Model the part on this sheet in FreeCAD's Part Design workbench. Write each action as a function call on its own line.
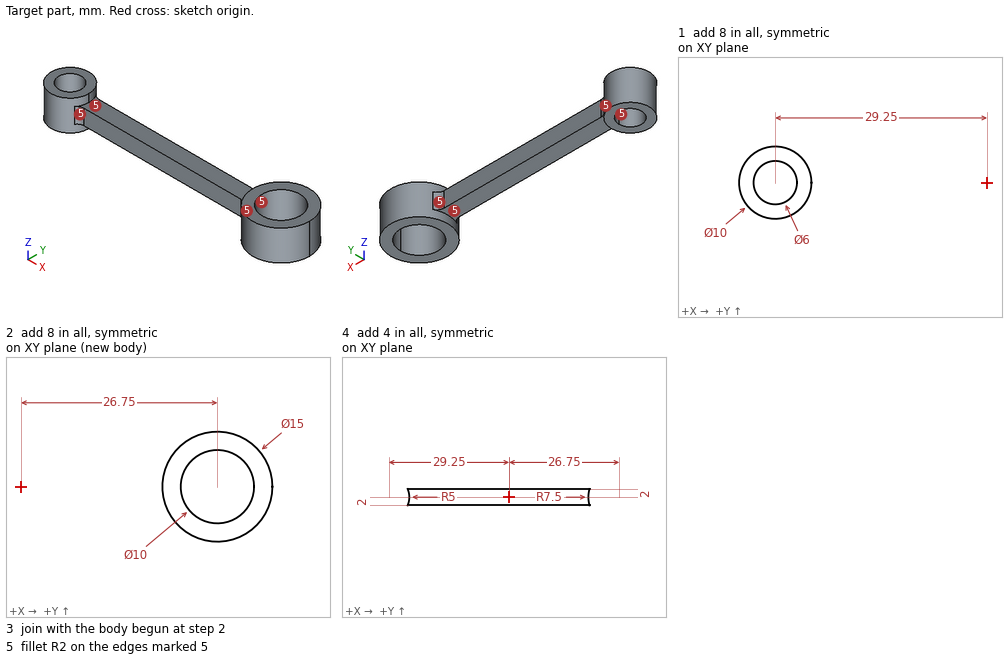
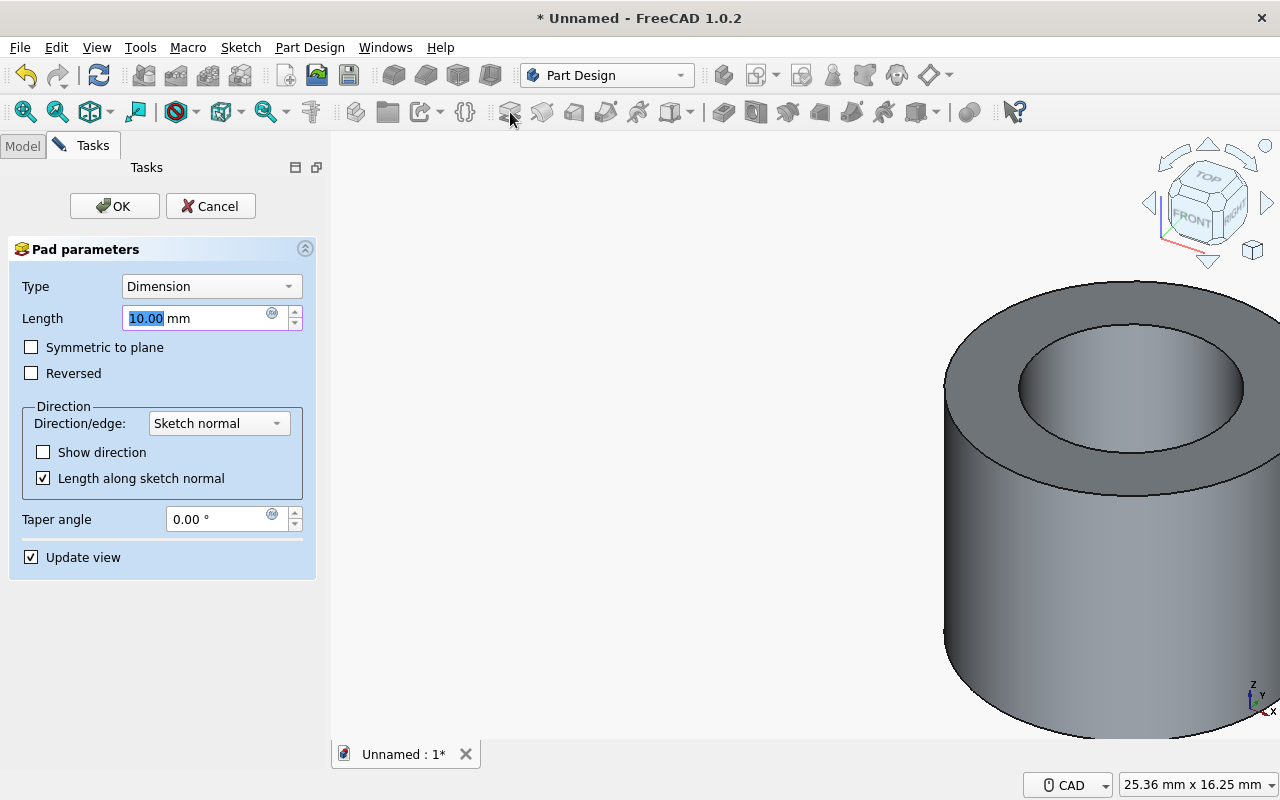
text(8)
key(Tab)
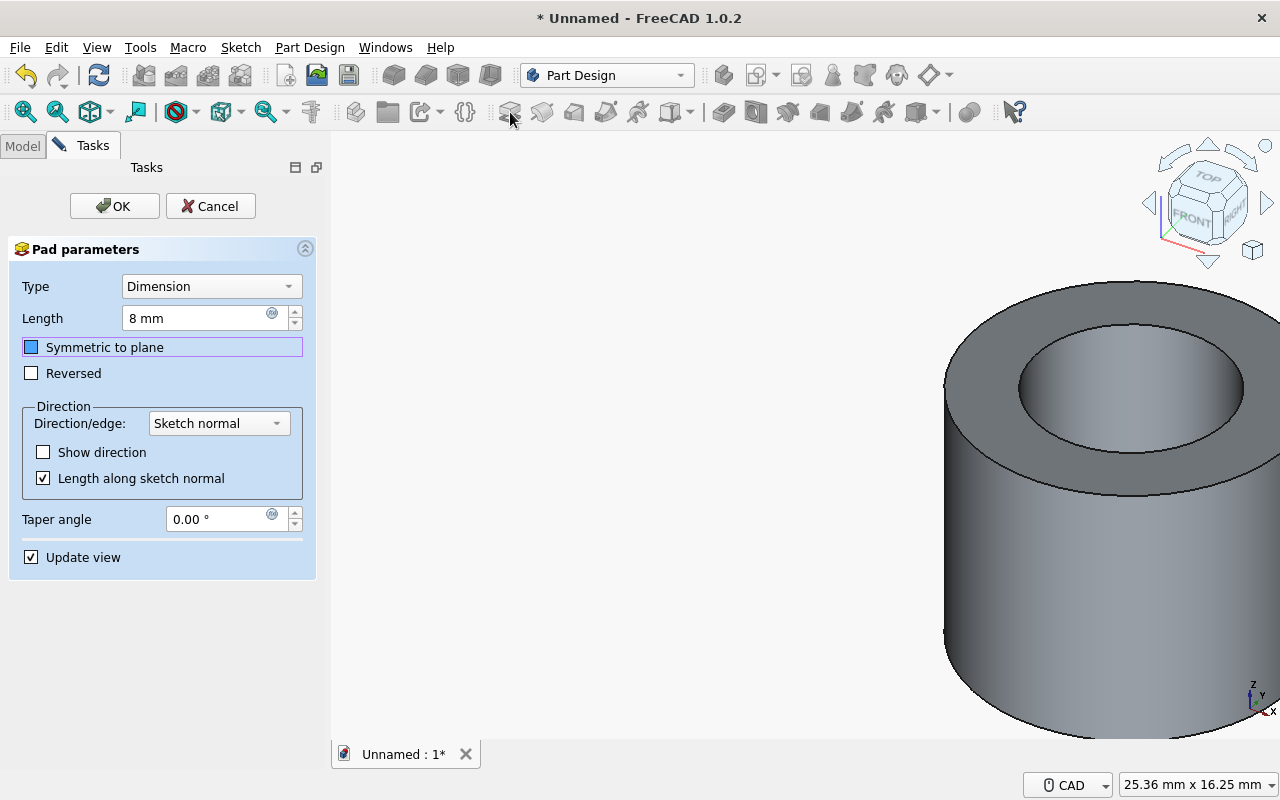
click(30, 347)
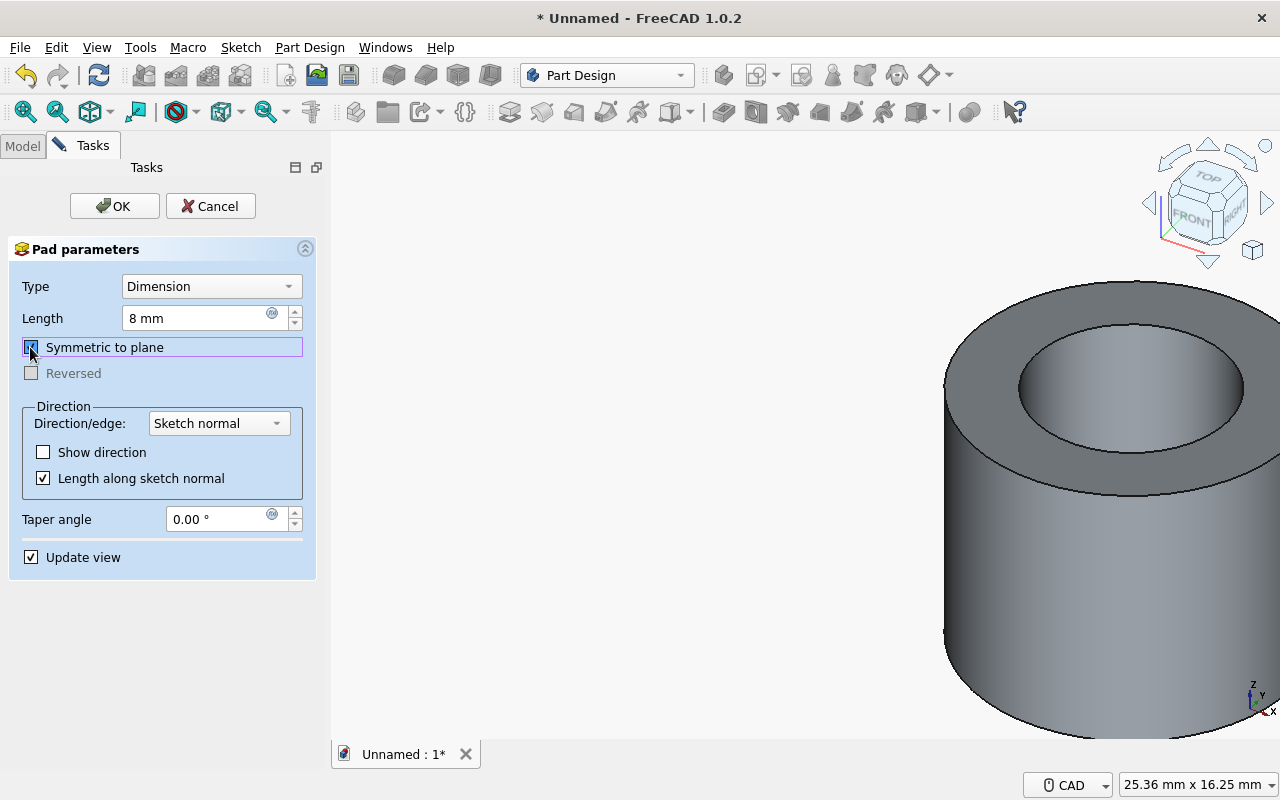
click(115, 206)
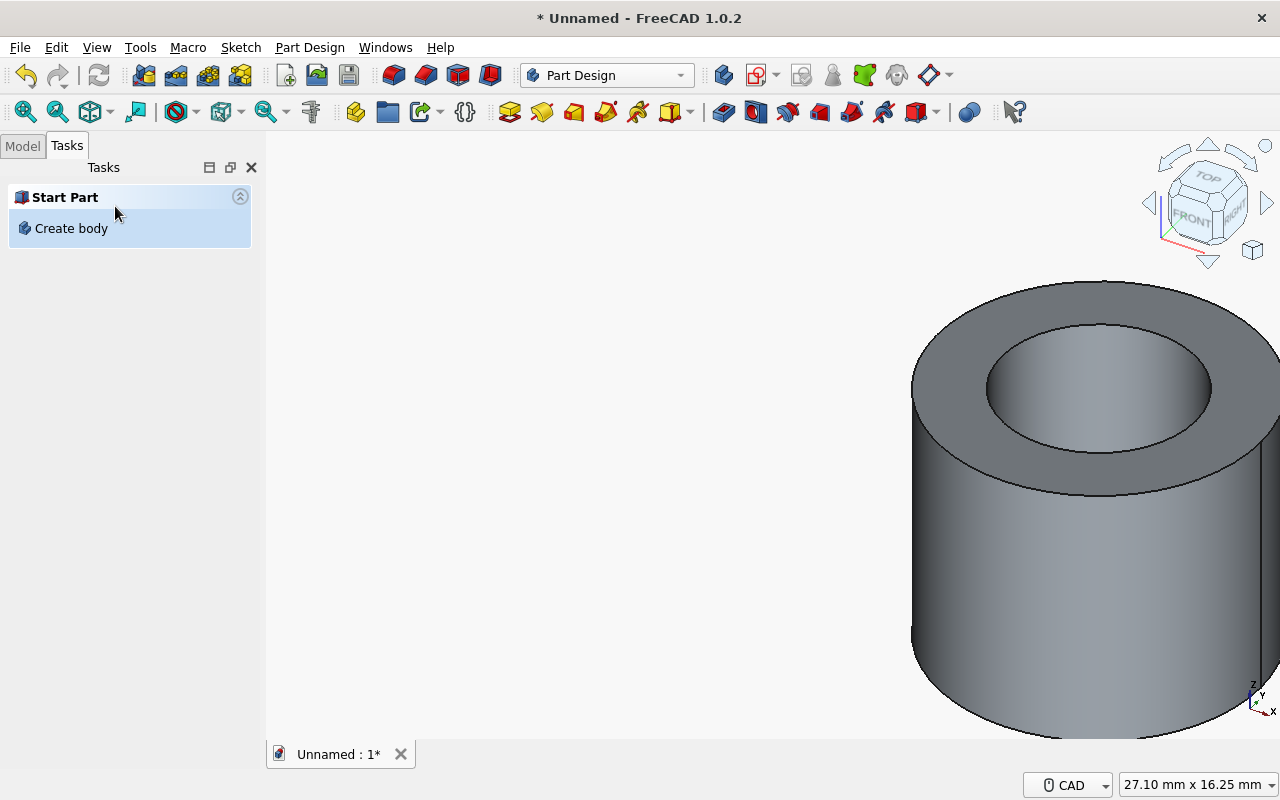
click(26, 112)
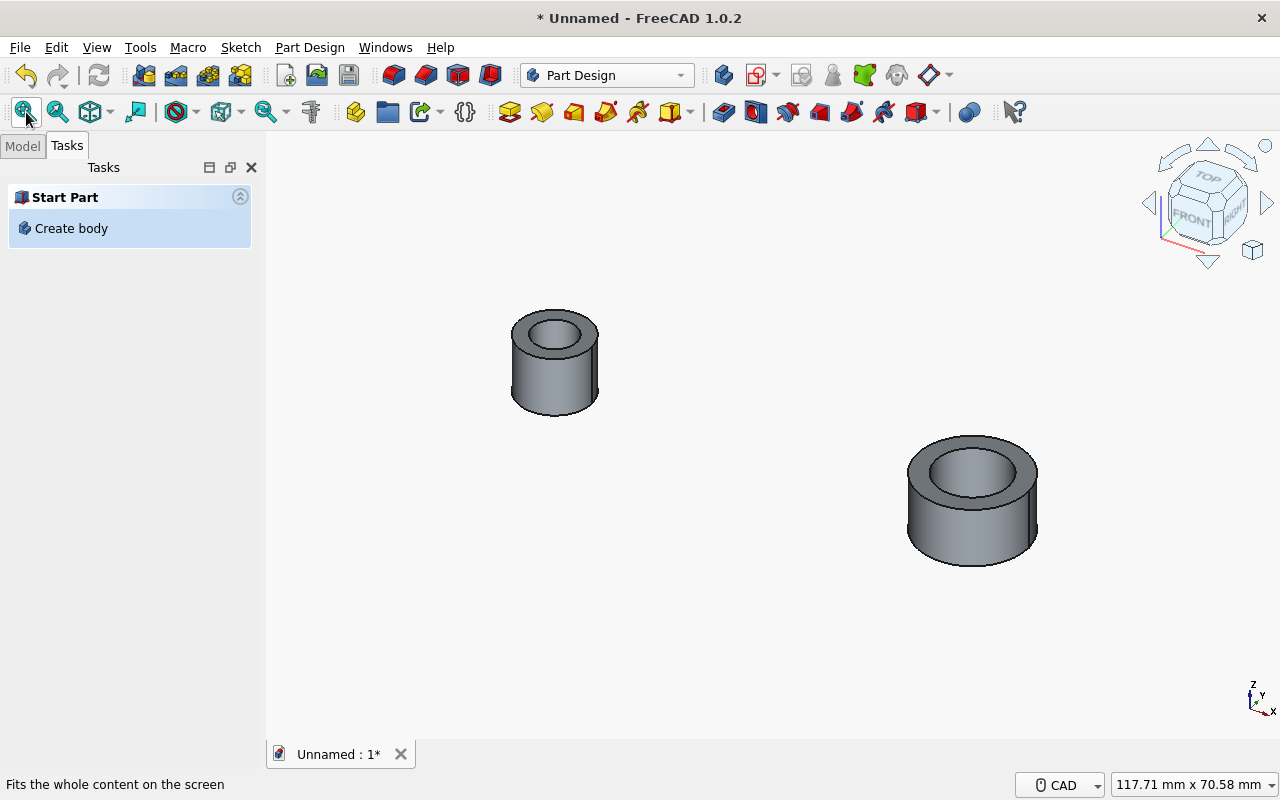
click(23, 145)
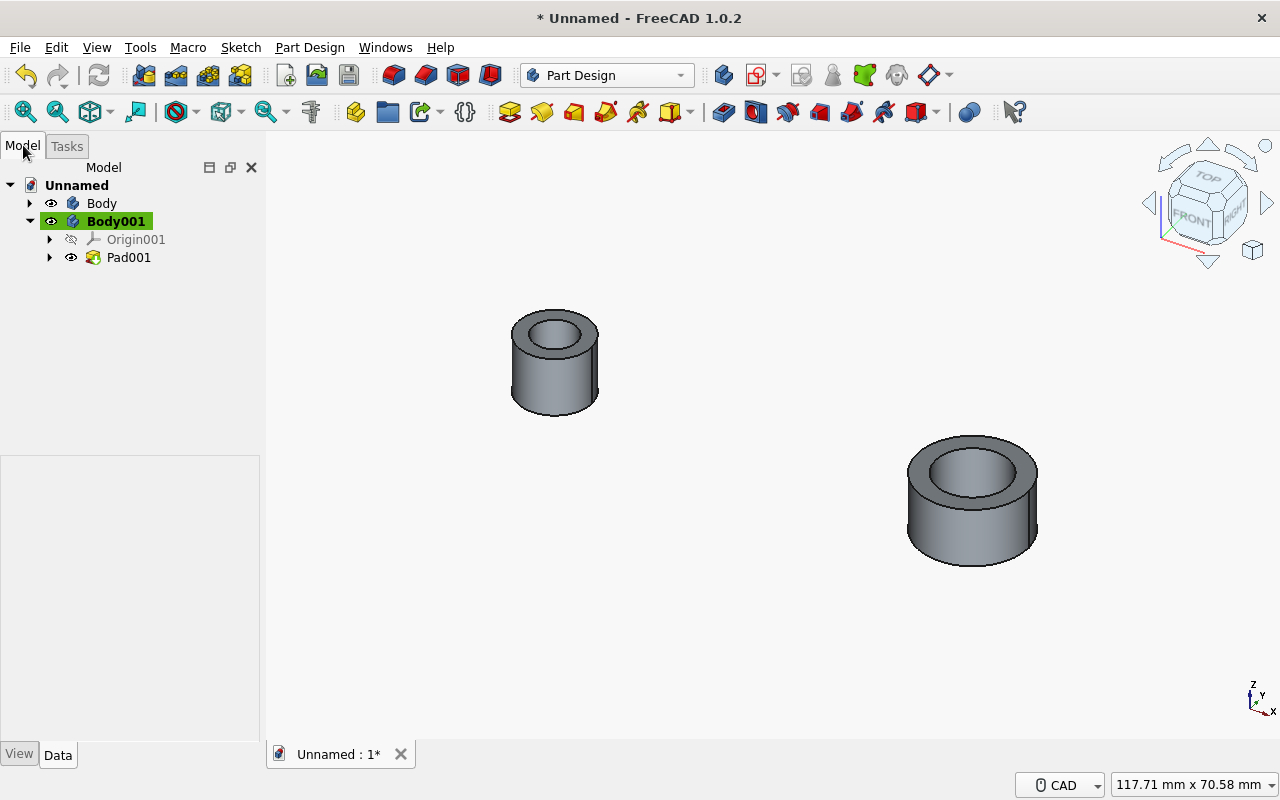
double_click(96, 203)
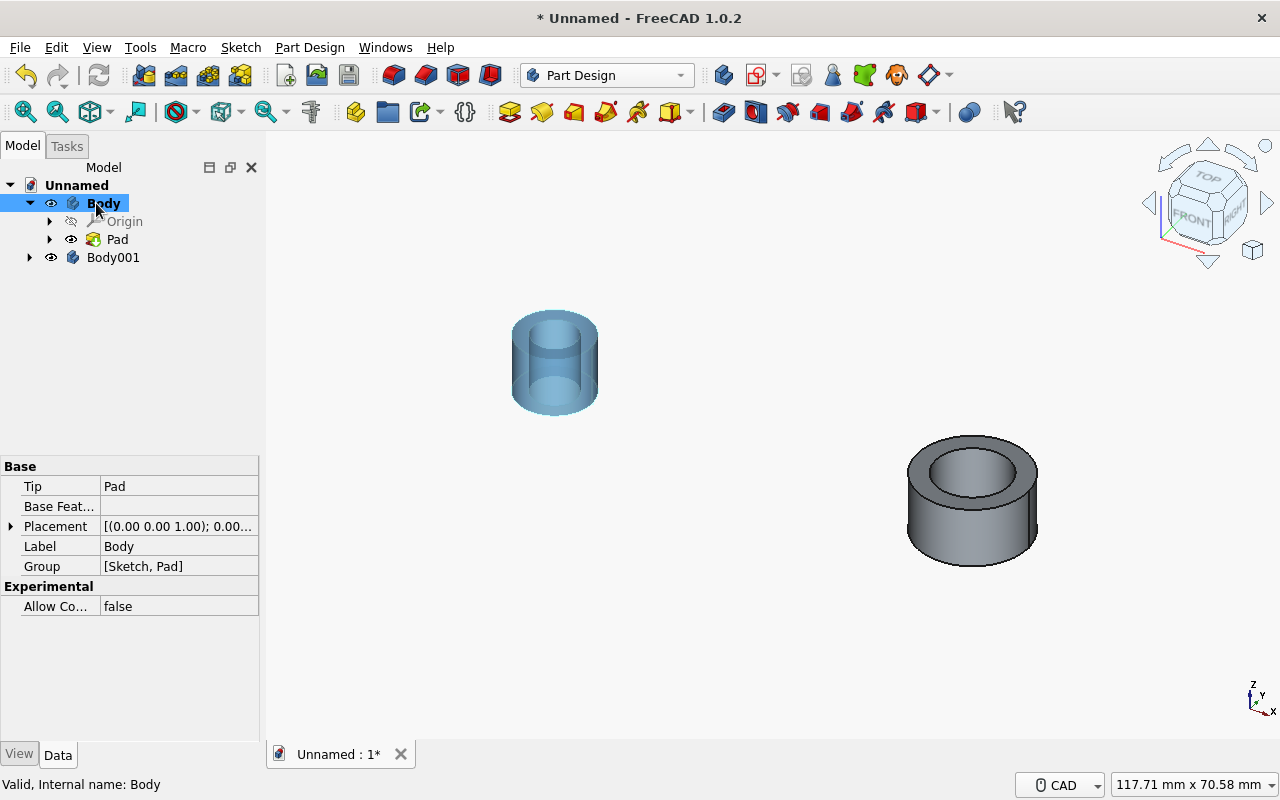
click(96, 203)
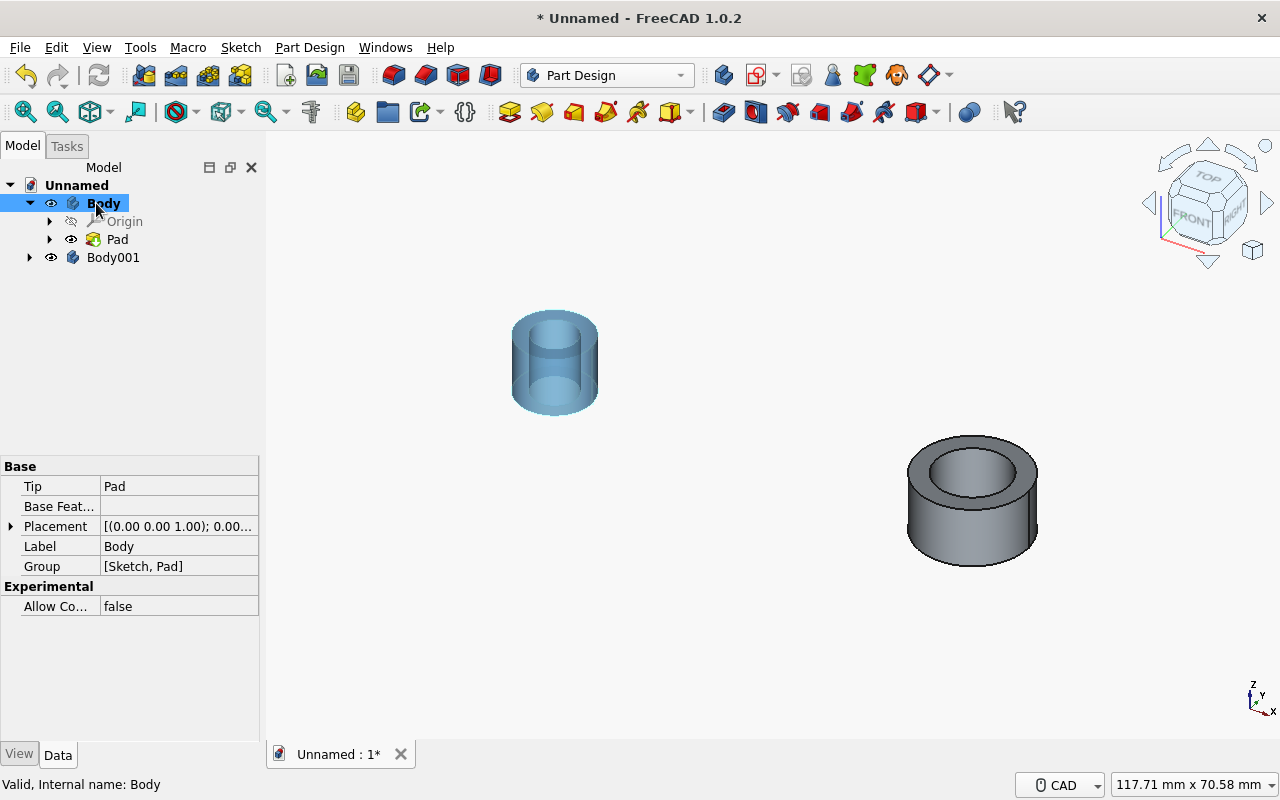
click(146, 606)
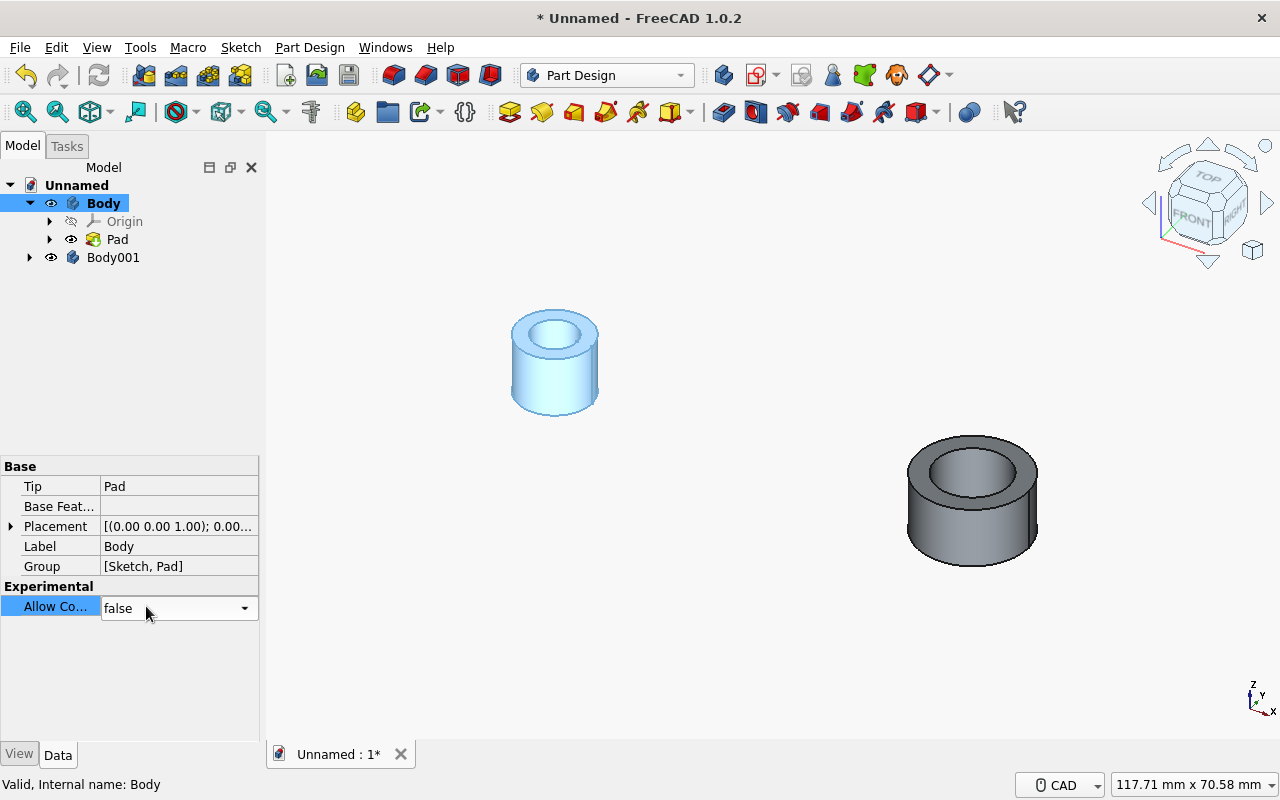
click(146, 606)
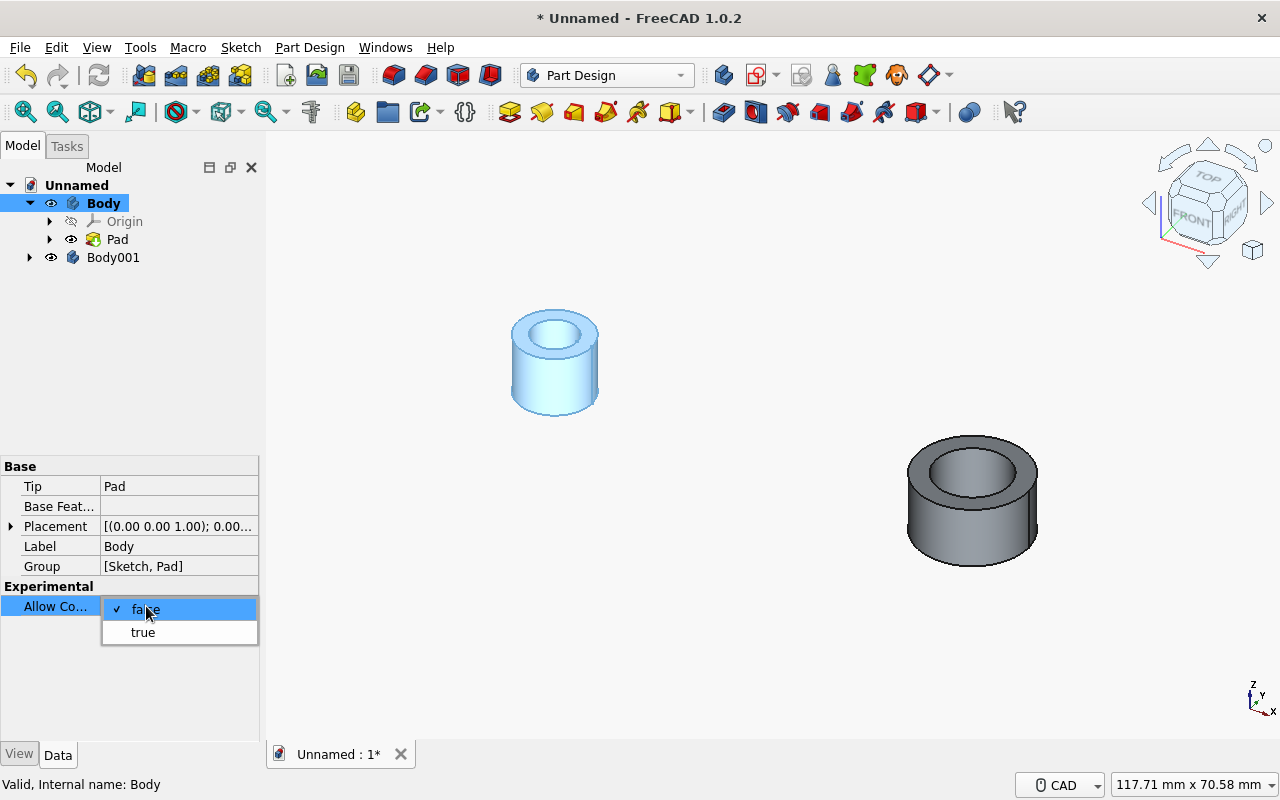
click(179, 632)
key(Return)